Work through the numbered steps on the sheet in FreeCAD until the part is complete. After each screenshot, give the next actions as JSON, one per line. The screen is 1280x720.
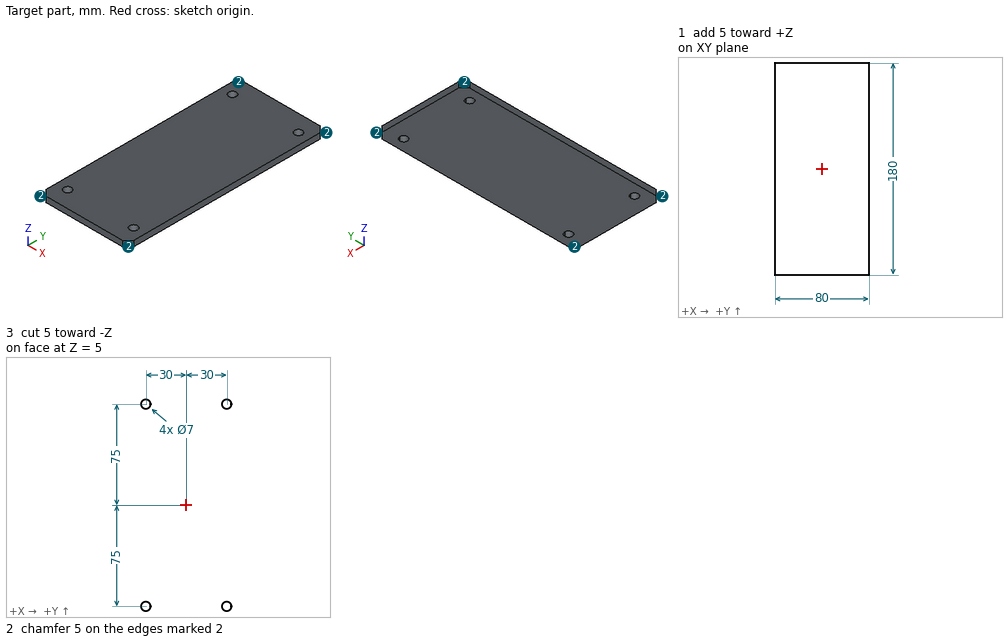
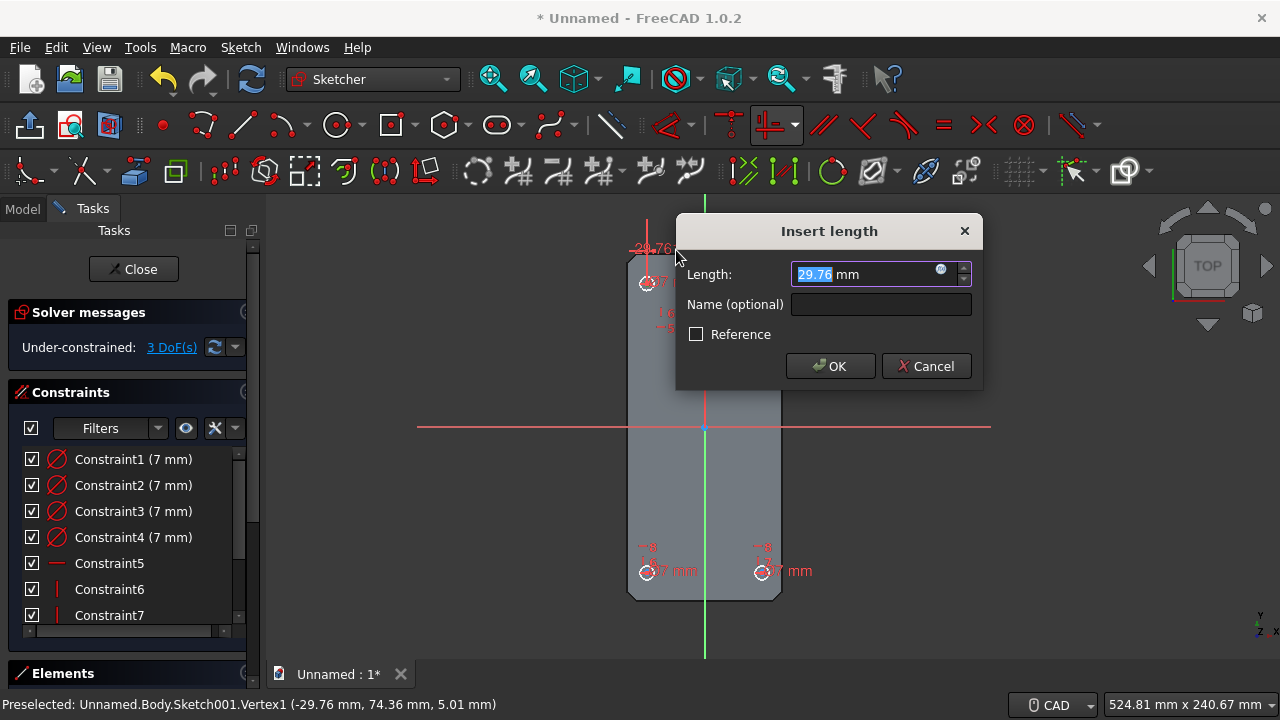
{"action": "type", "text": "30"}
{"action": "key", "text": "Return"}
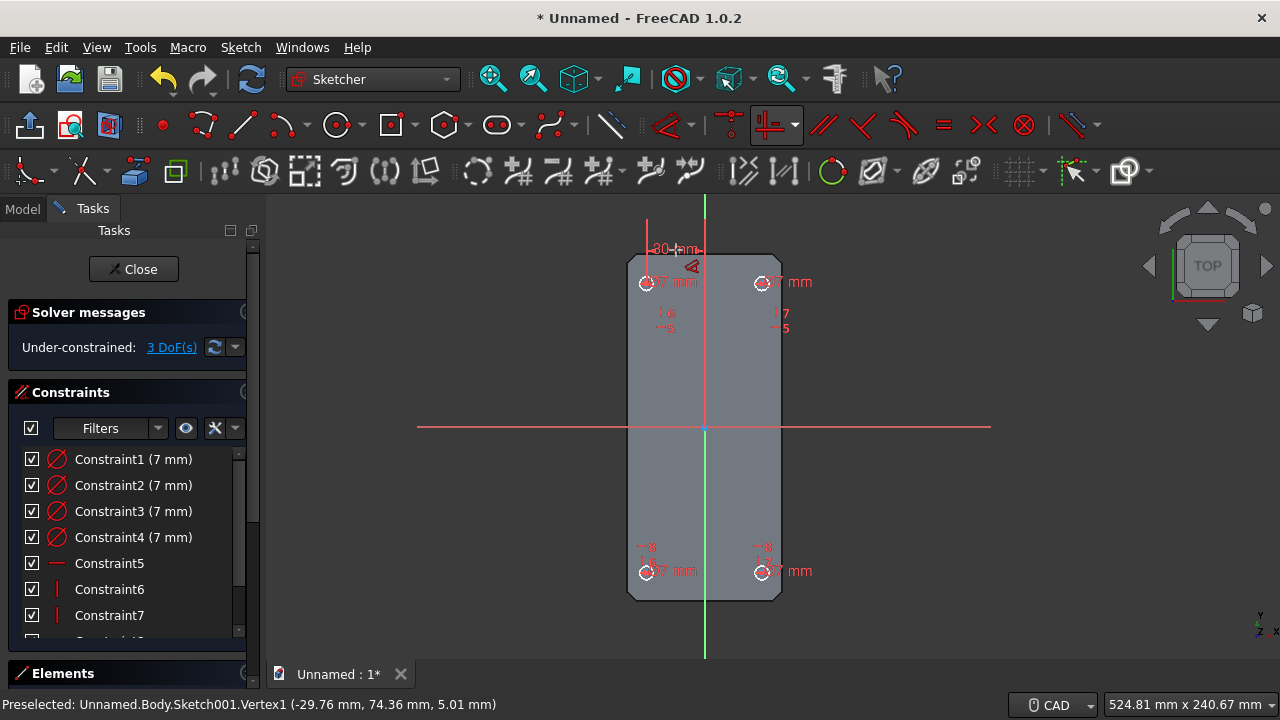
{"action": "left_click", "coordinate": [647, 284]}
{"action": "left_click", "coordinate": [613, 356]}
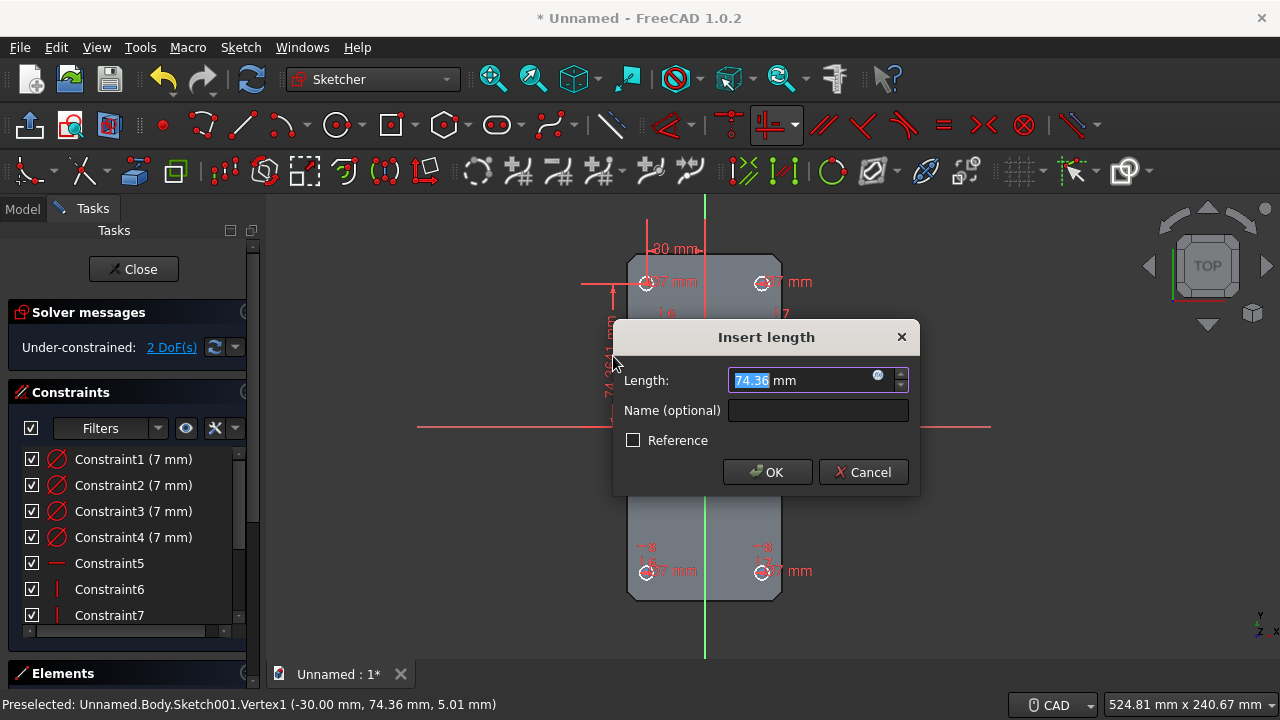
{"action": "type", "text": "75"}
{"action": "key", "text": "Return"}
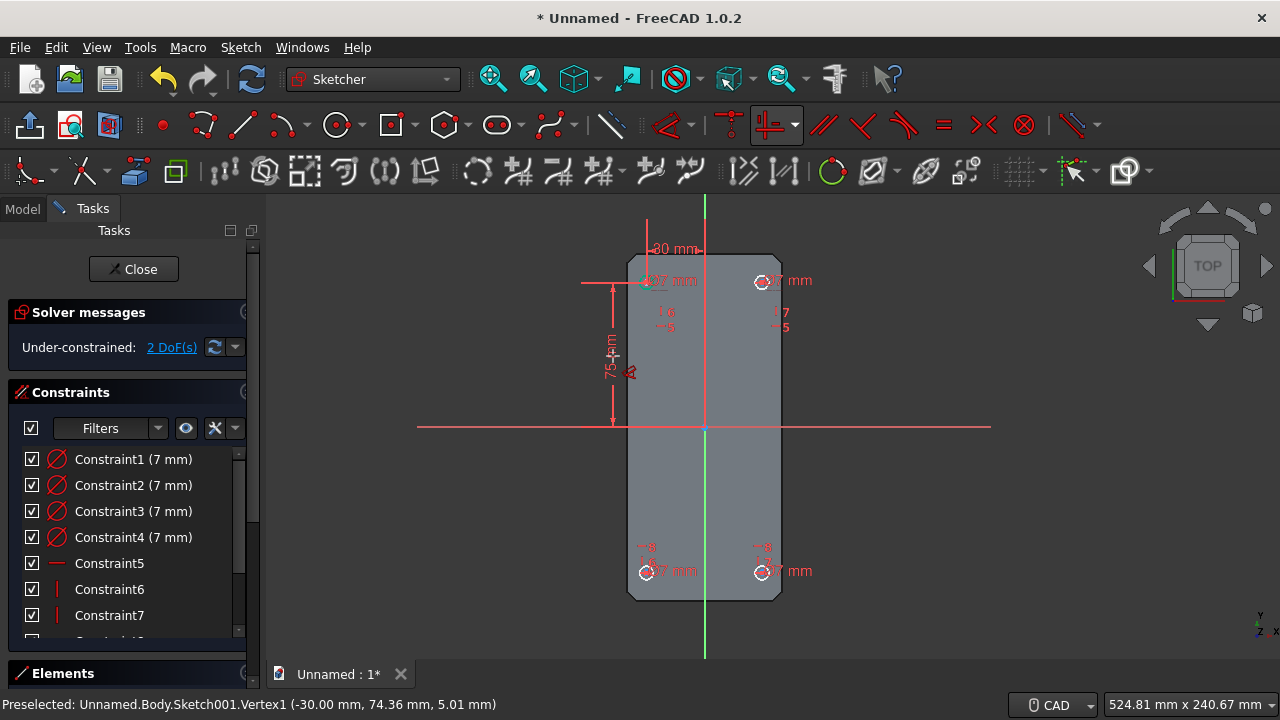
{"action": "left_click", "coordinate": [762, 283]}
{"action": "left_click", "coordinate": [746, 249]}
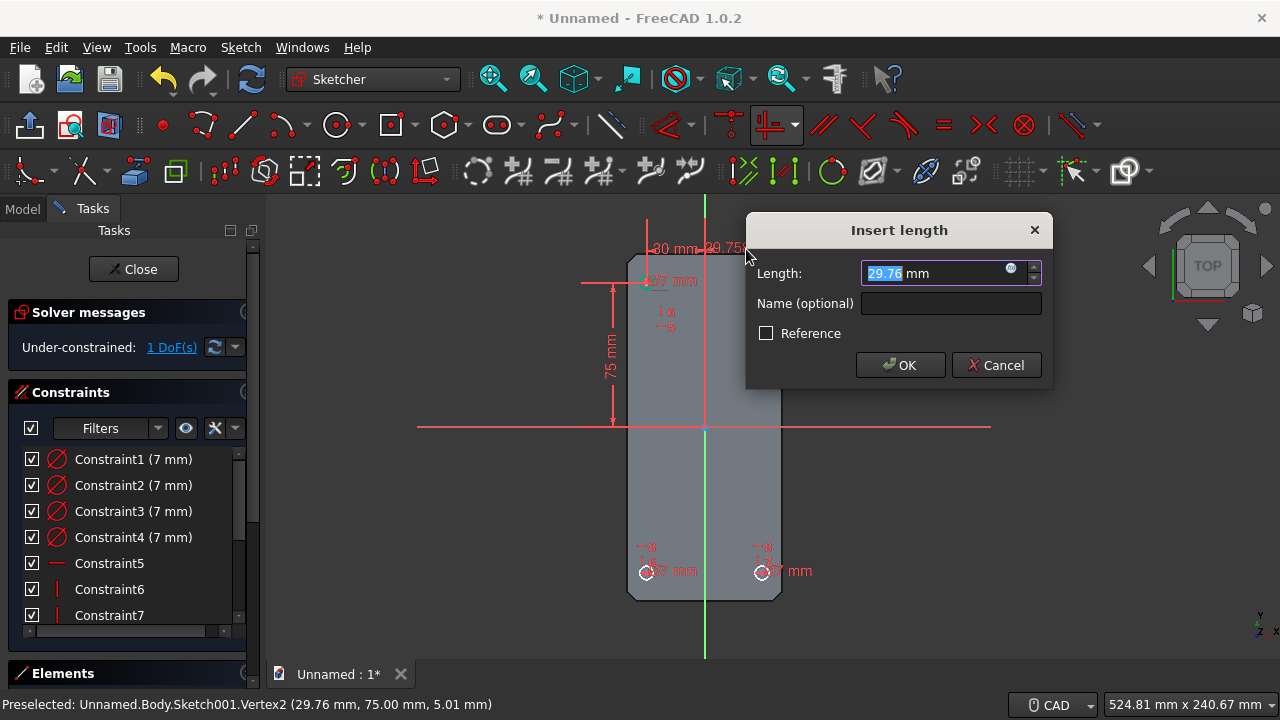
{"action": "type", "text": "30"}
{"action": "key", "text": "Return"}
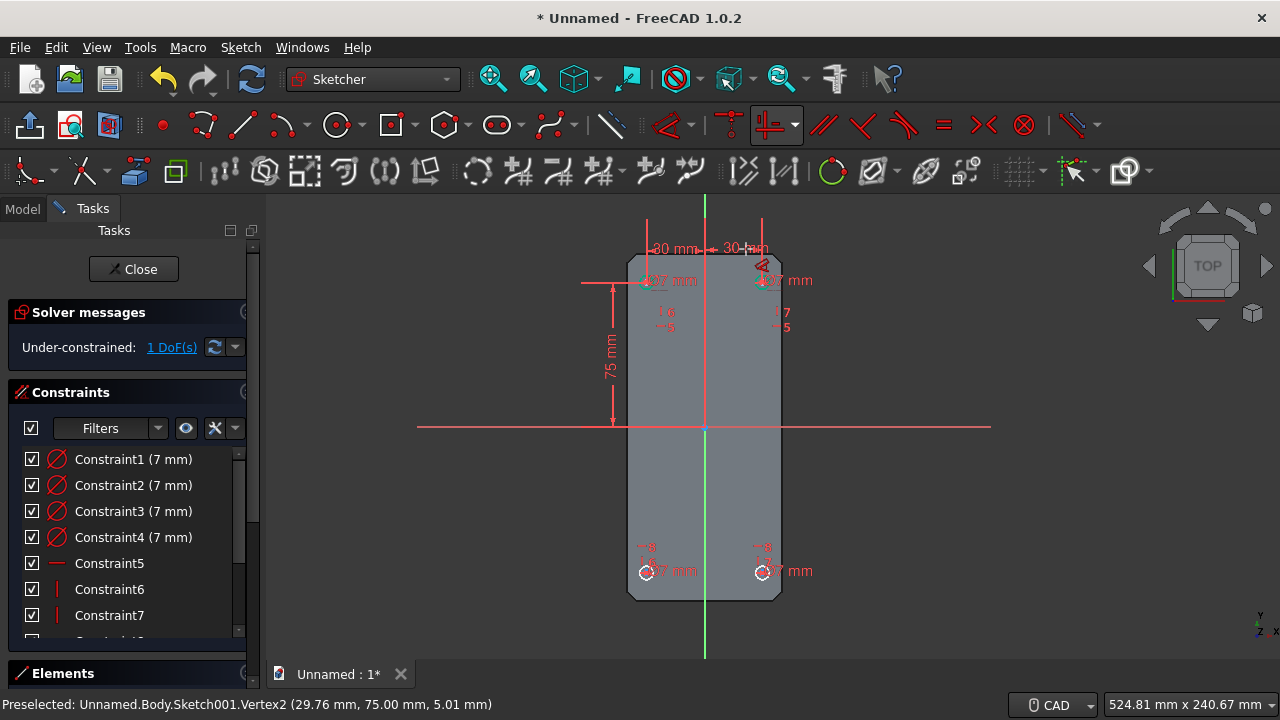
{"action": "left_click", "coordinate": [647, 573]}
{"action": "left_click", "coordinate": [613, 500]}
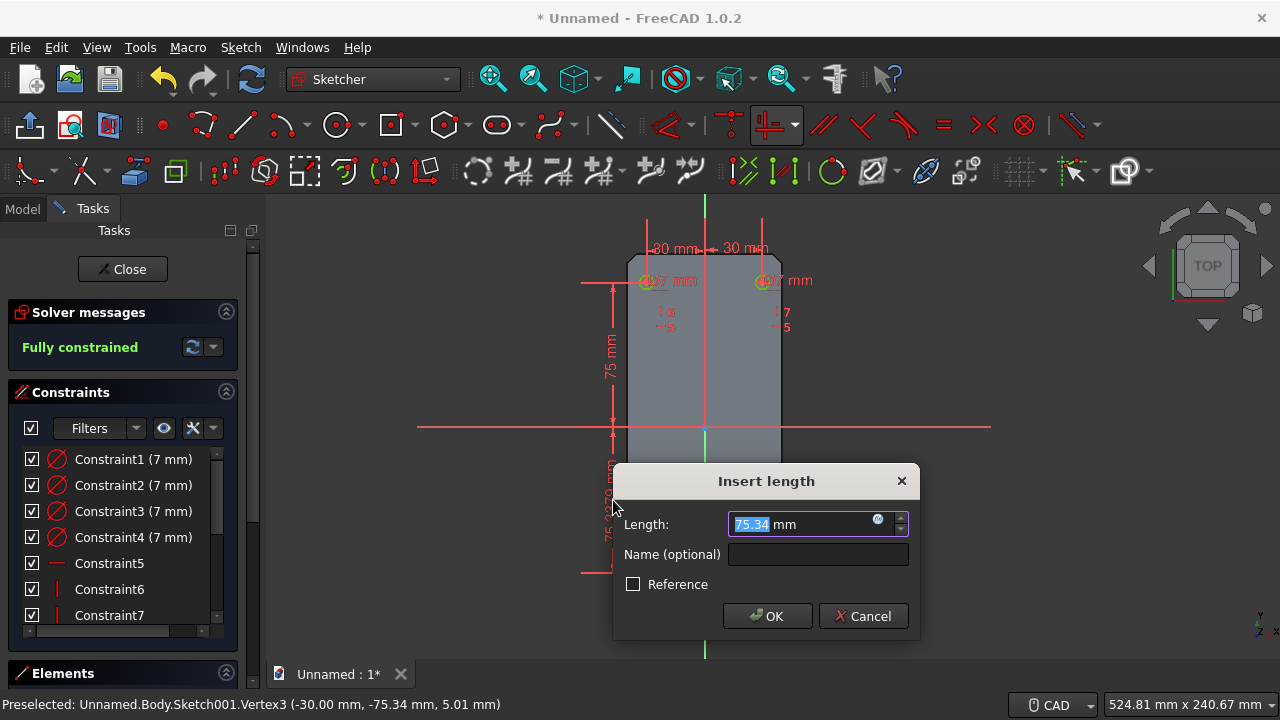
{"action": "type", "text": "75"}
{"action": "key", "text": "Return"}
{"action": "key", "text": "Escape"}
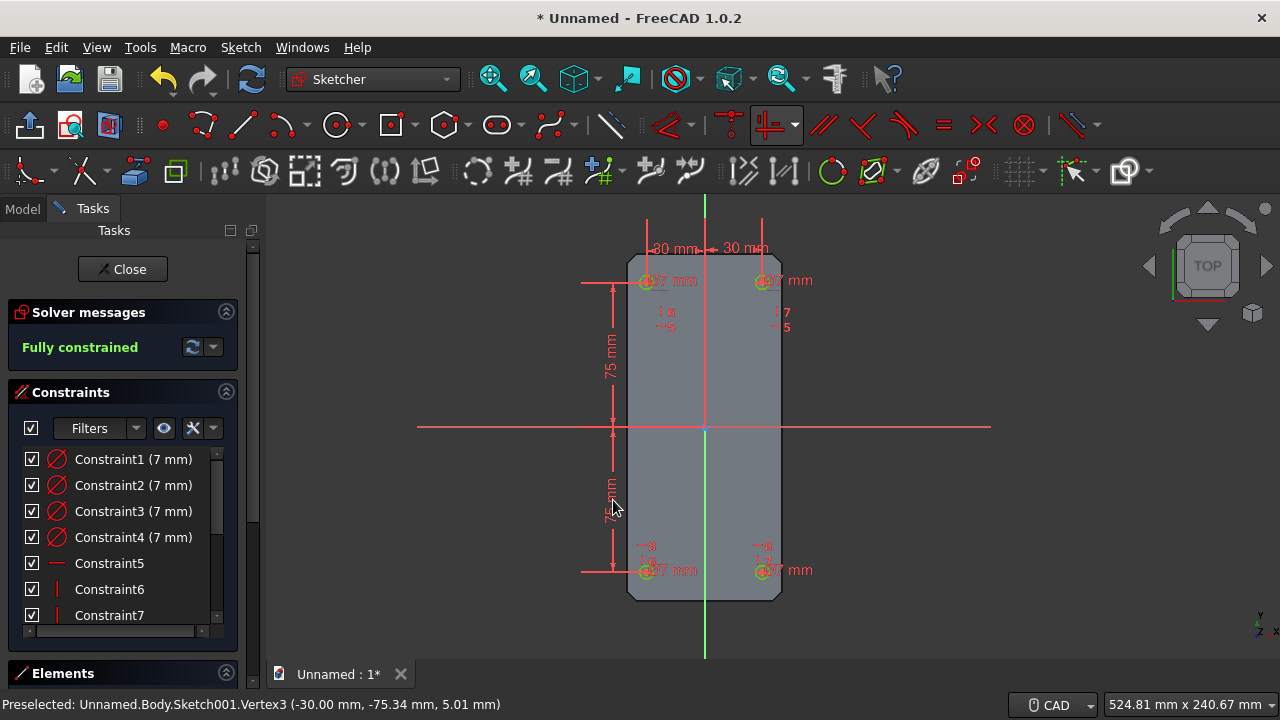
{"action": "left_click", "coordinate": [123, 269]}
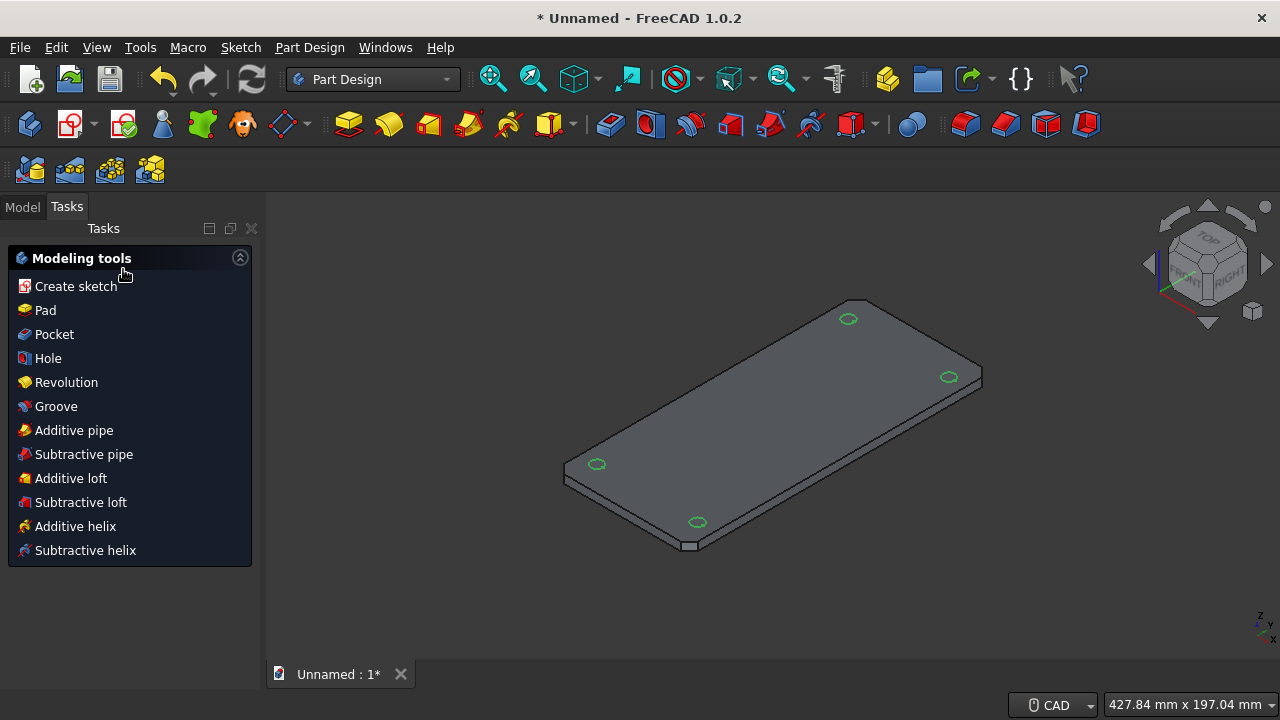
{"action": "left_click", "coordinate": [612, 124]}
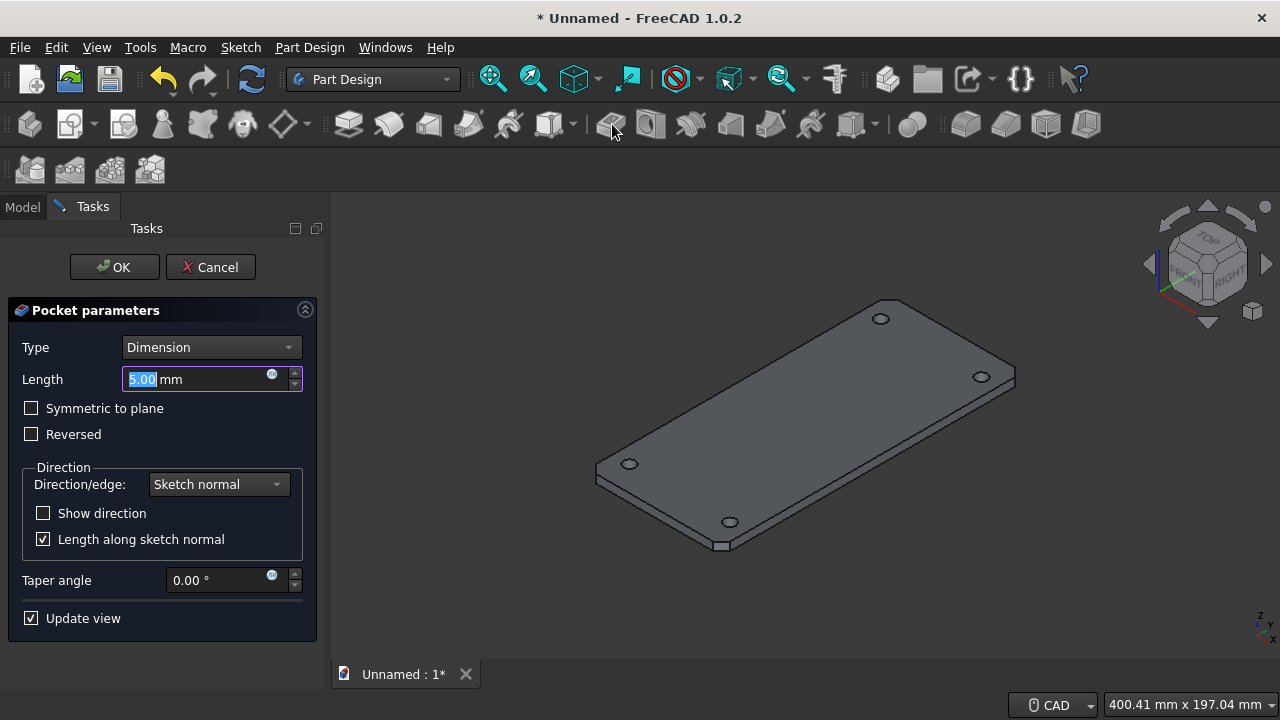
{"action": "type", "text": "5"}
{"action": "key", "text": "Tab"}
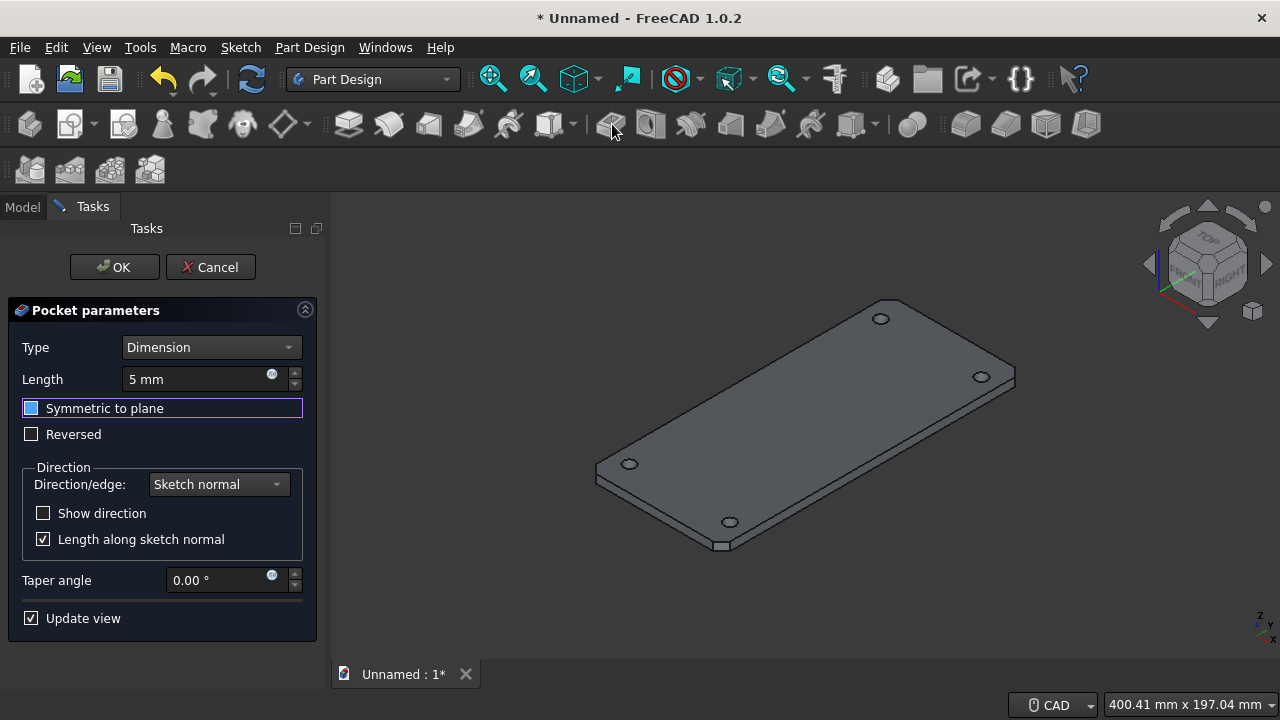
{"action": "left_click", "coordinate": [115, 267]}